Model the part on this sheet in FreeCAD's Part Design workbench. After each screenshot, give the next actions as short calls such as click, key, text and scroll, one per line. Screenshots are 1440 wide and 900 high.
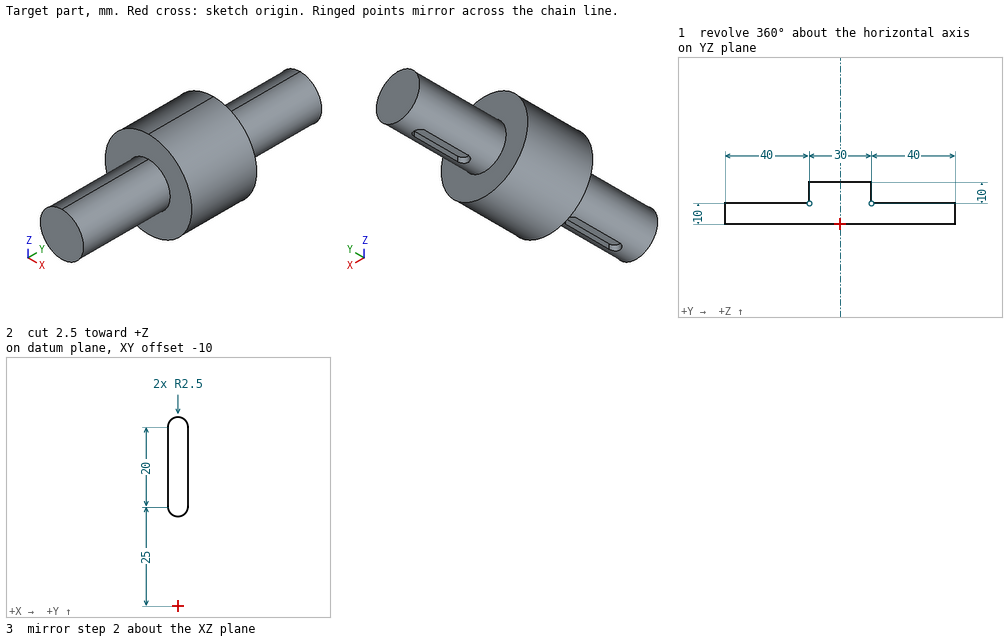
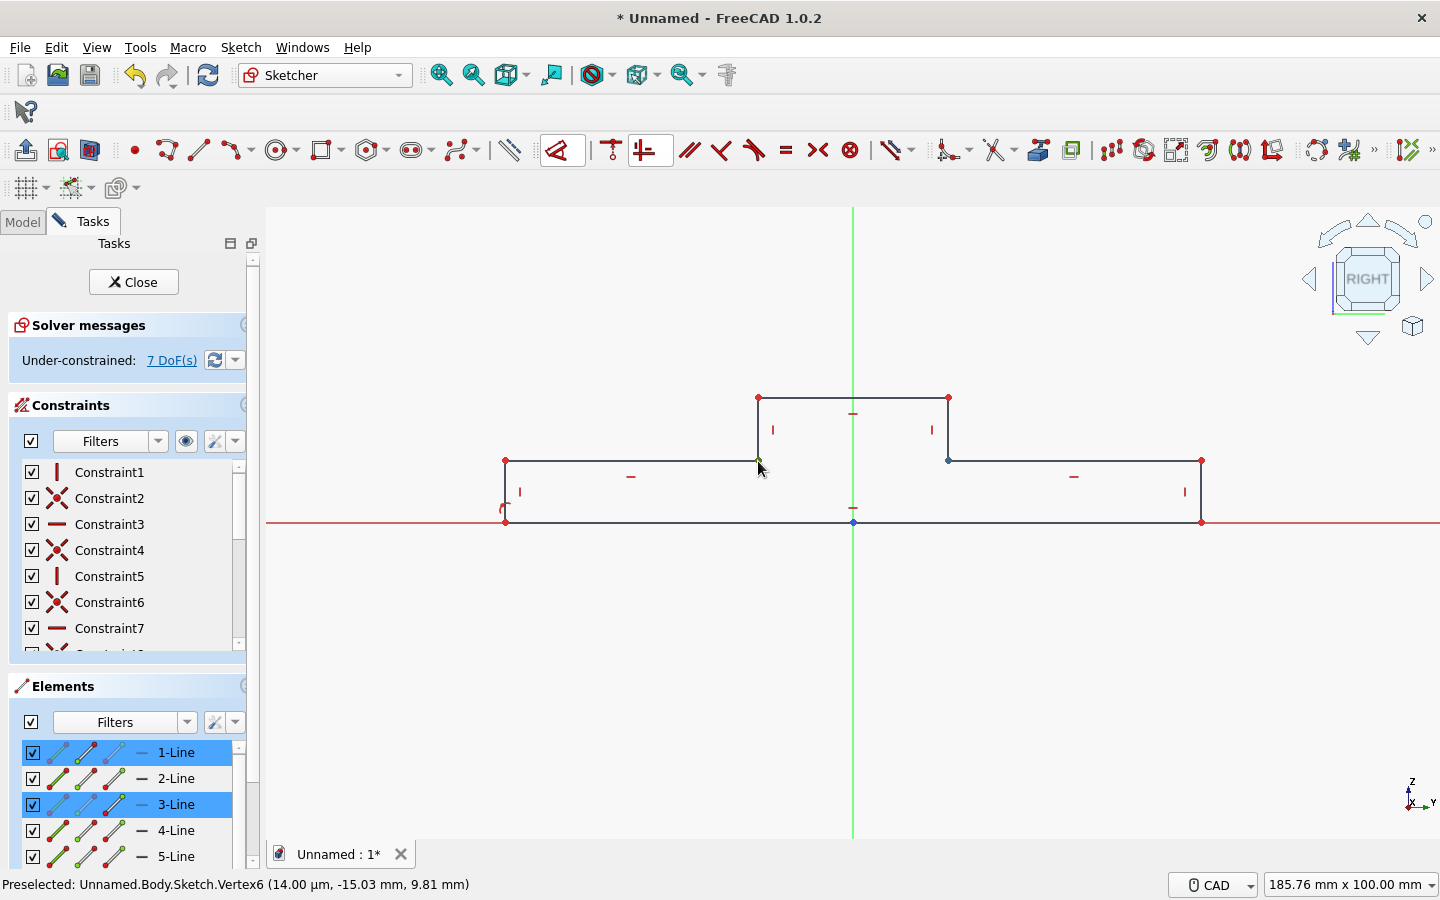
click(853, 770)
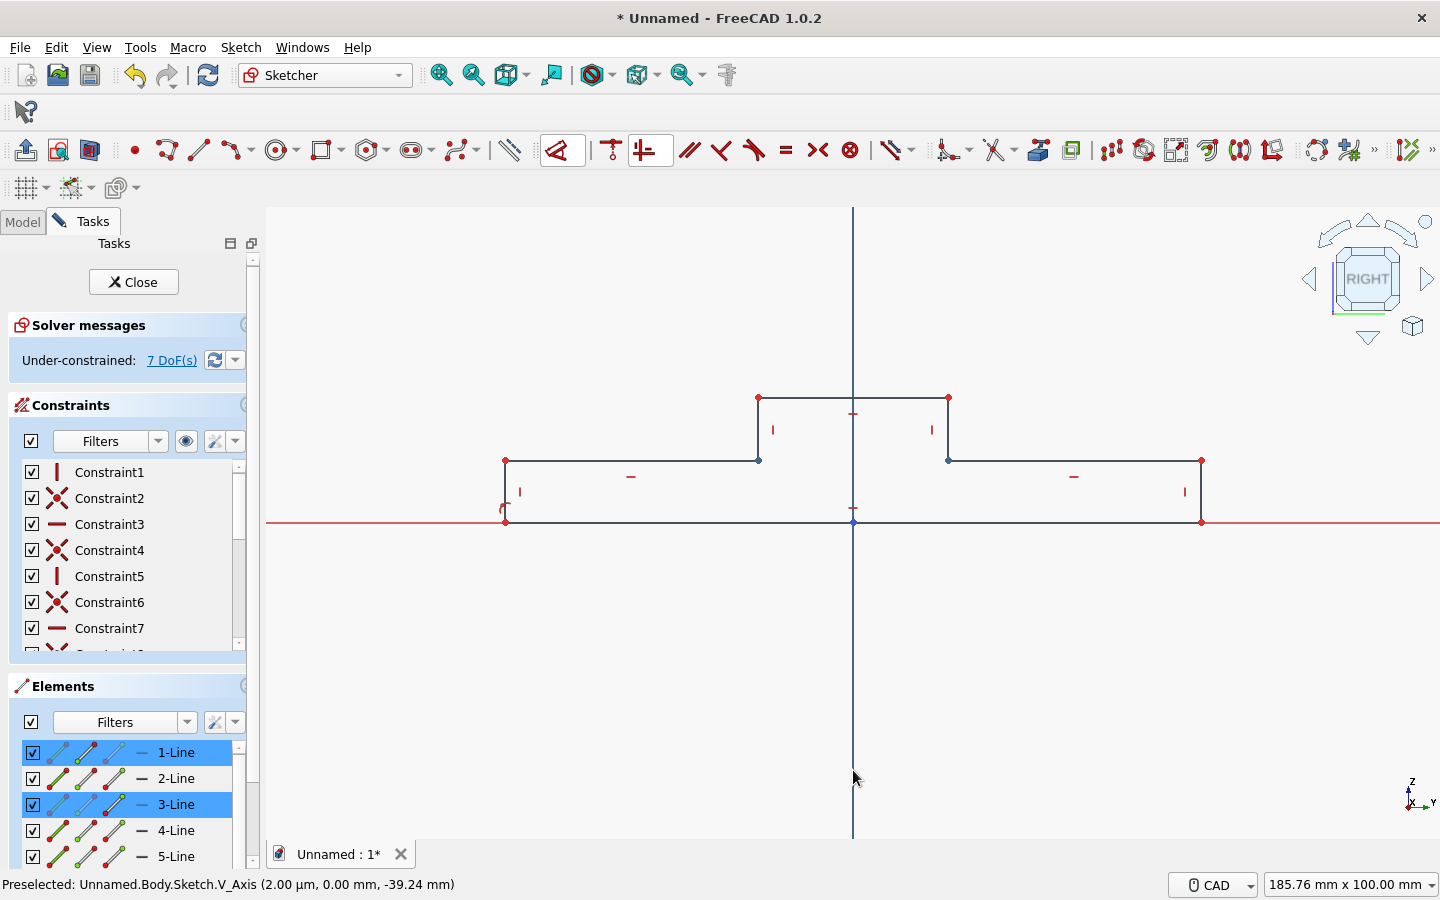
click(818, 150)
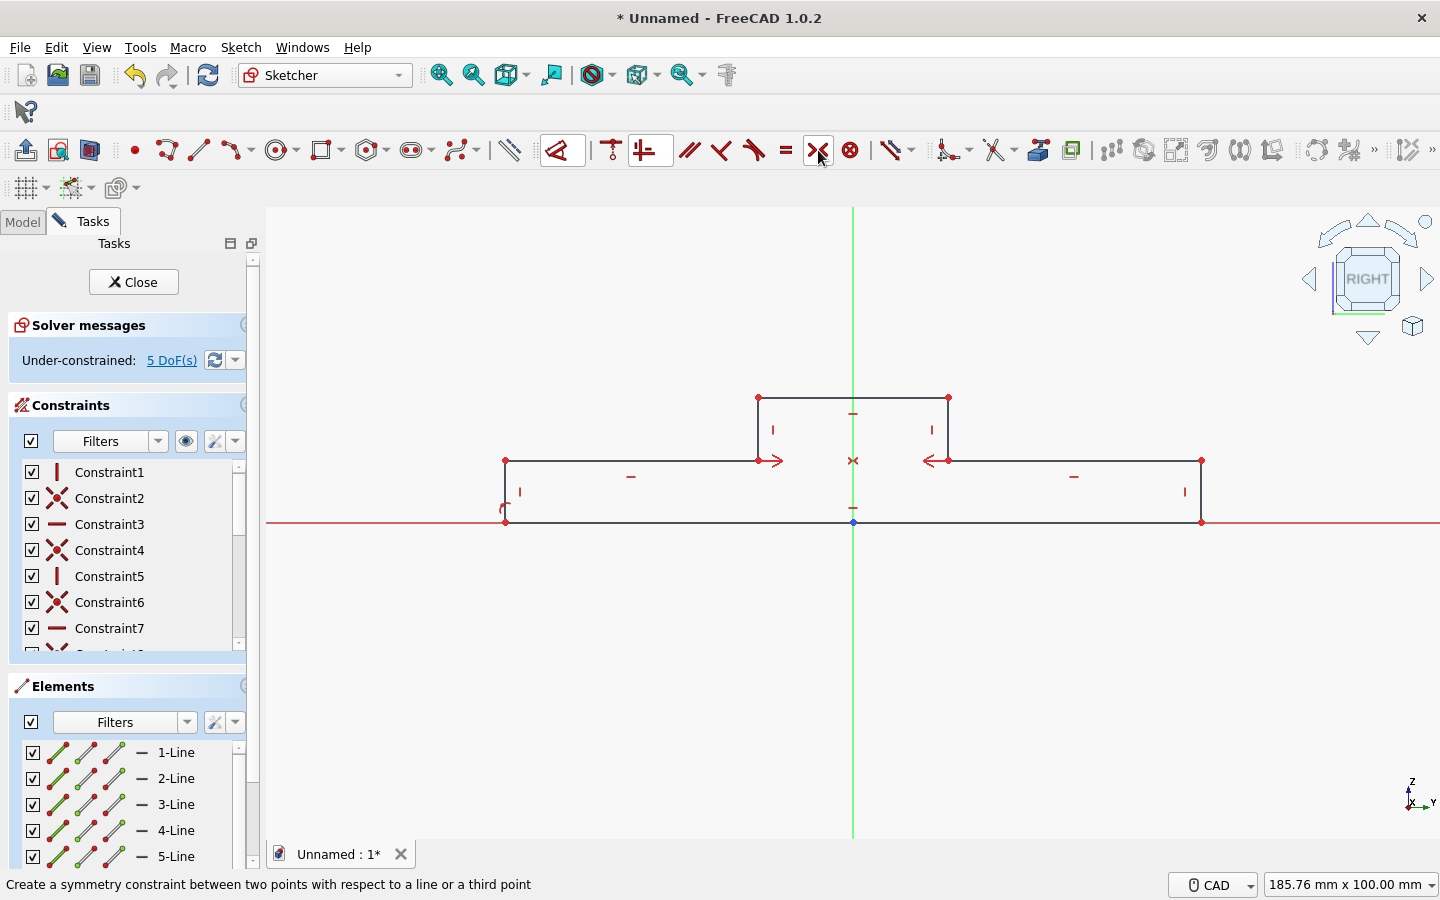
click(556, 150)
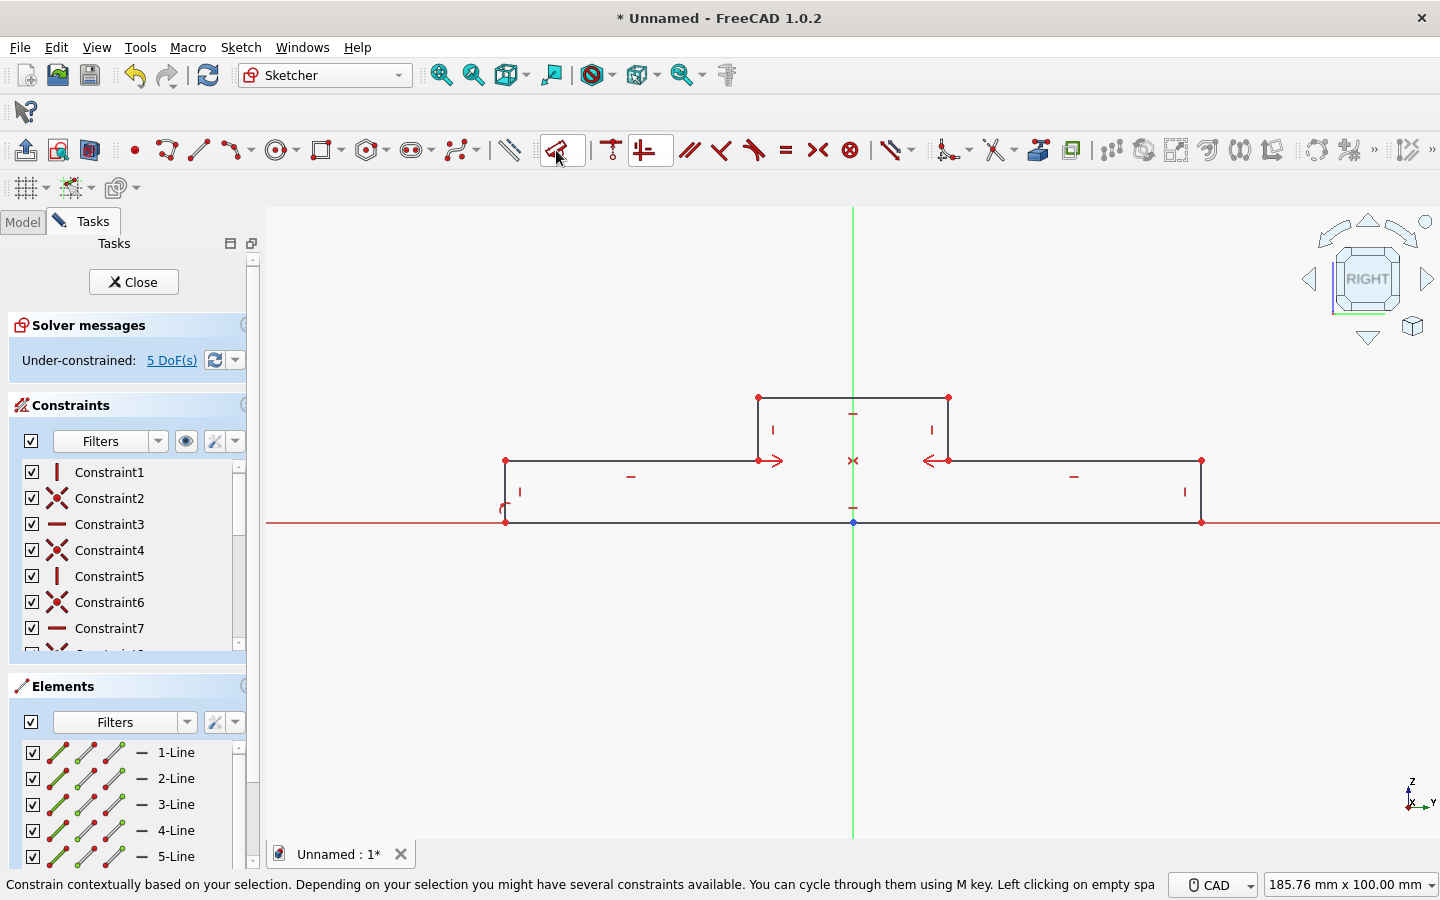
click(948, 442)
click(982, 430)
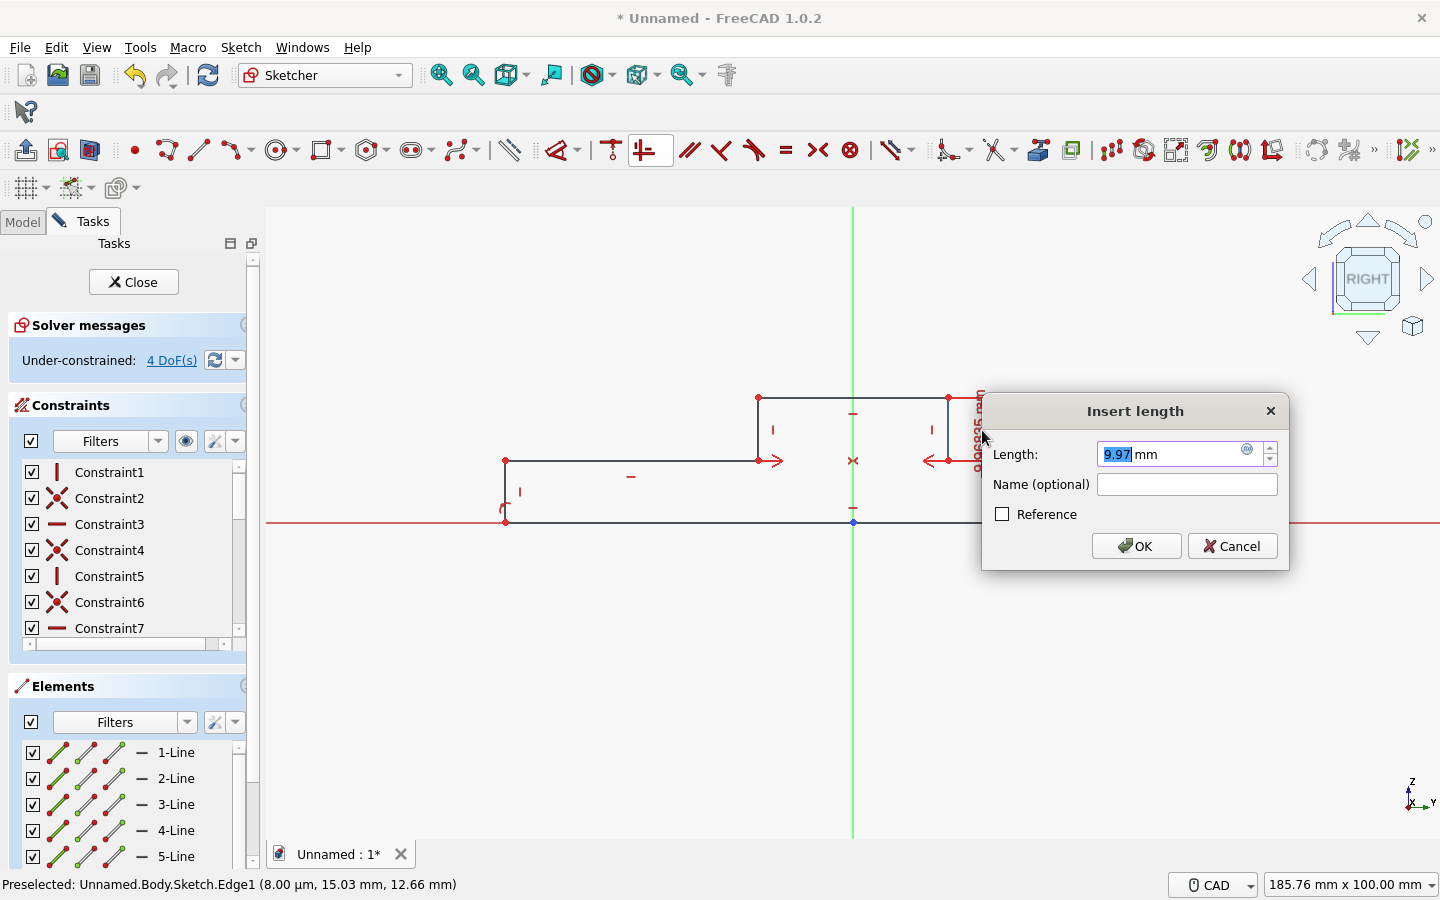
text(10)
key(Return)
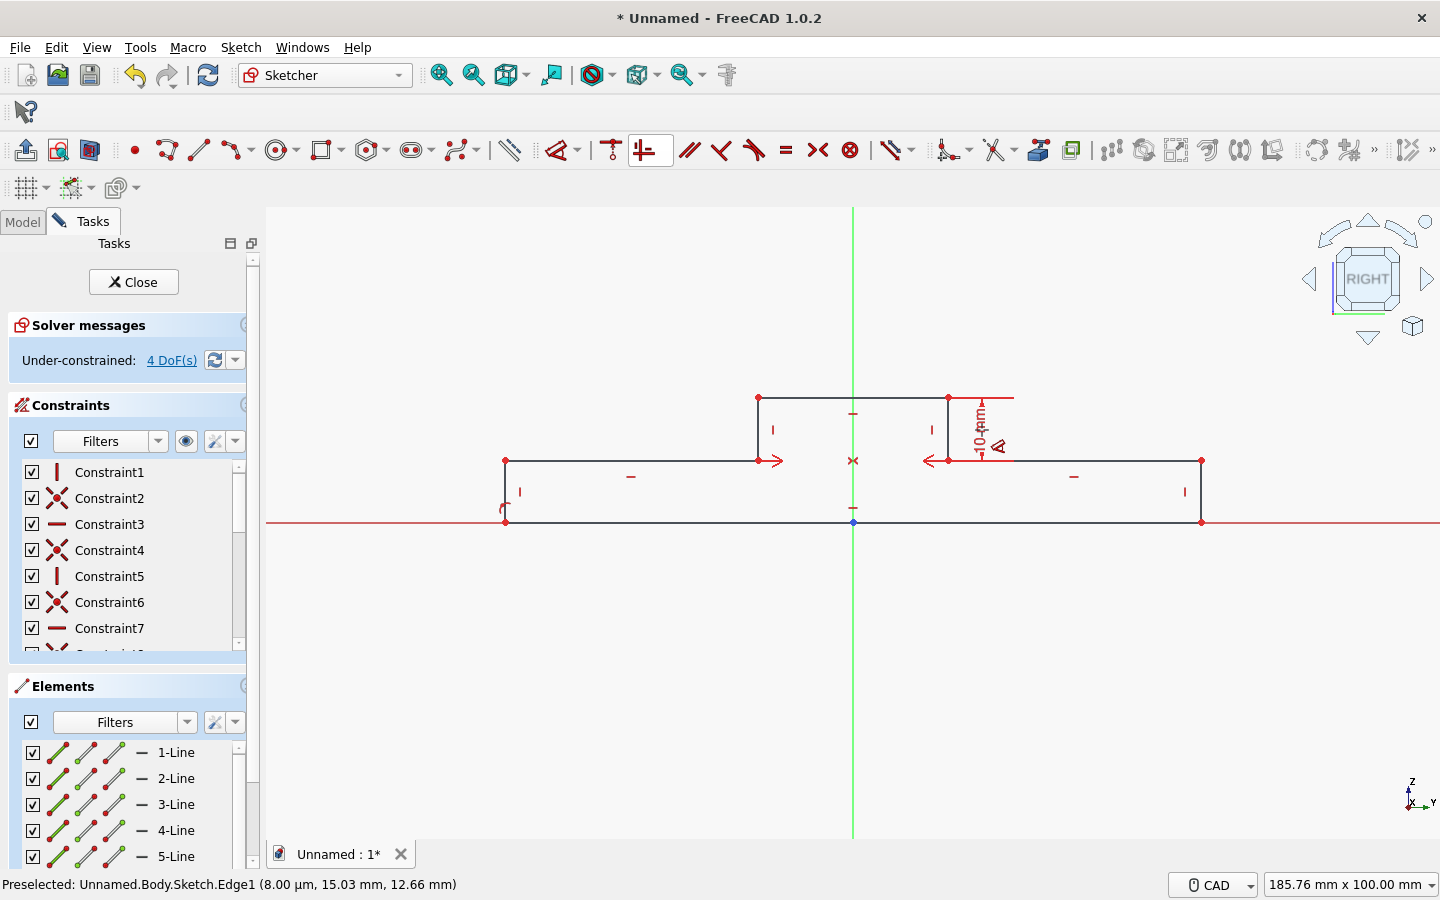
click(891, 398)
click(809, 364)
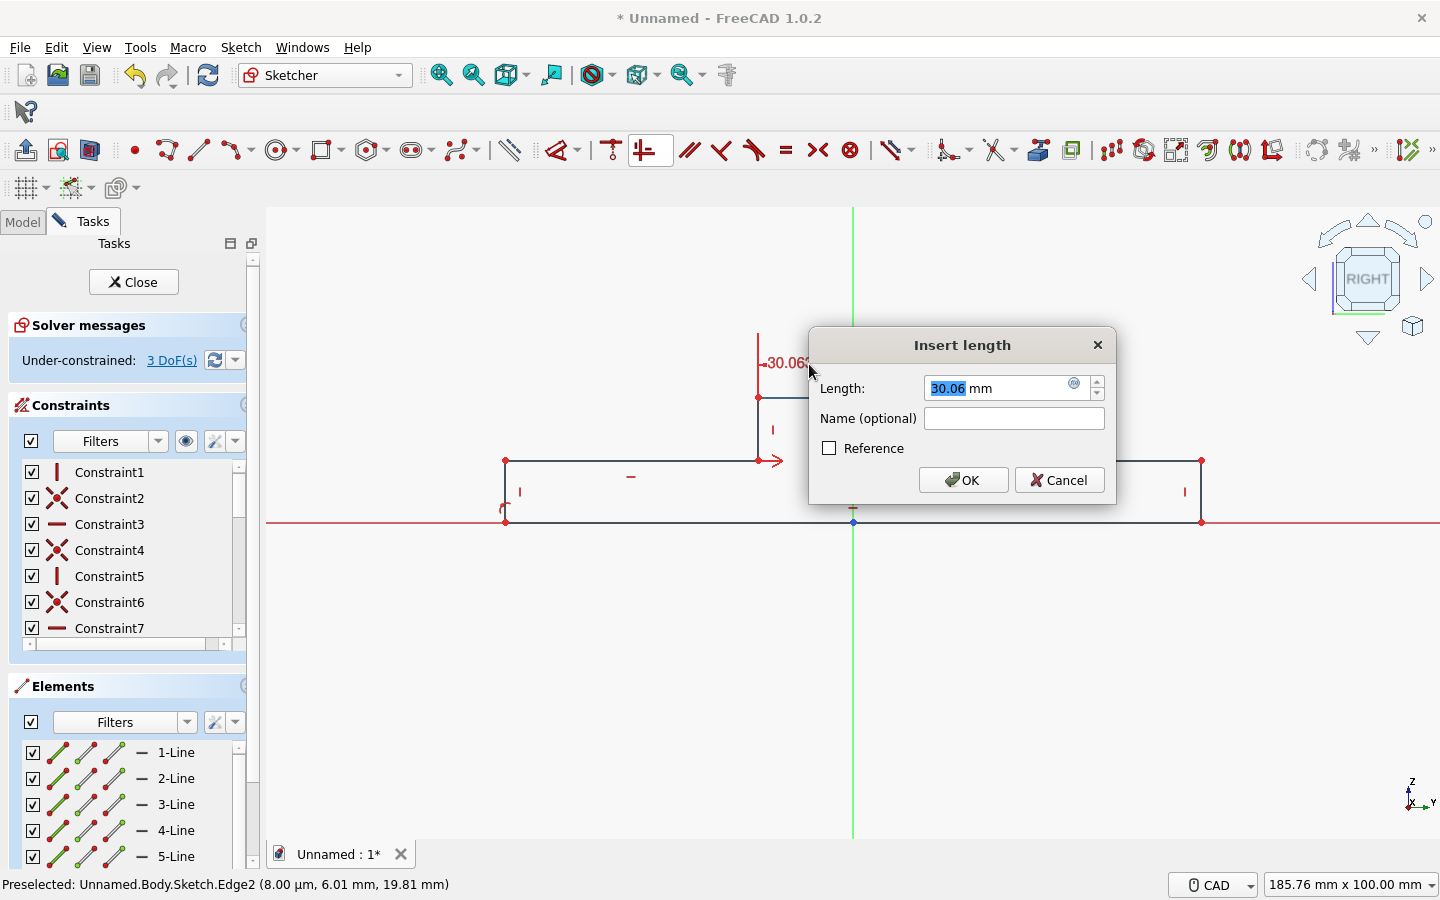
text(30)
key(Return)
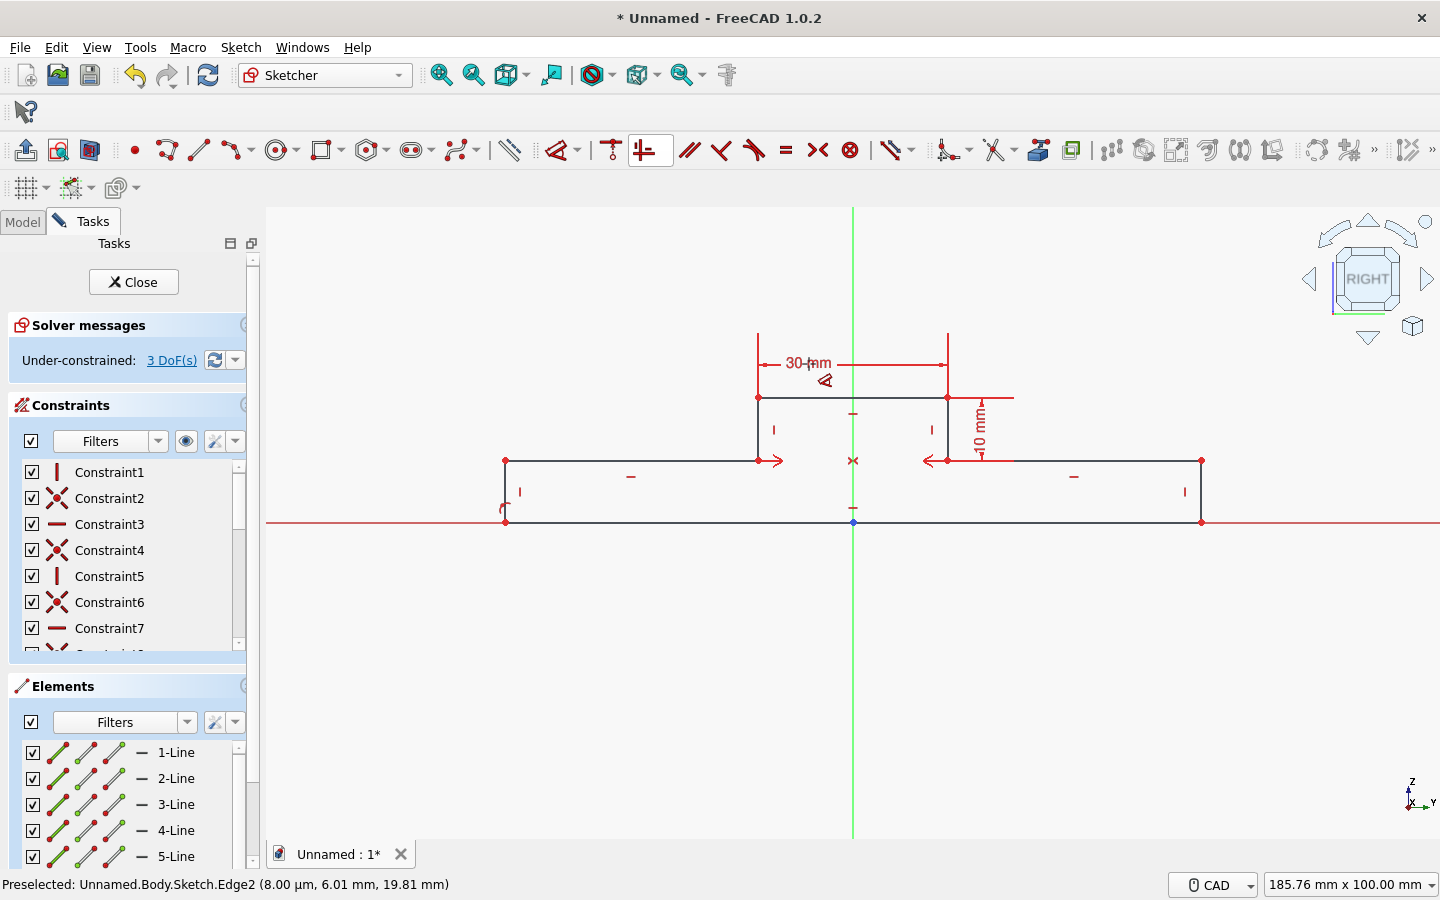
click(682, 461)
click(632, 495)